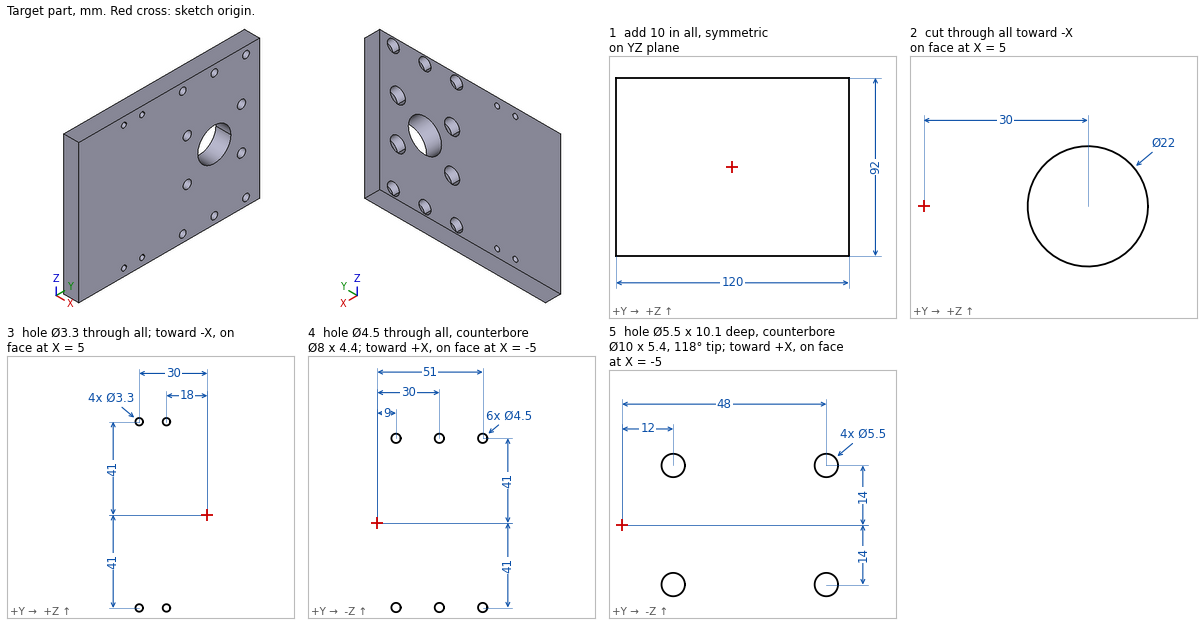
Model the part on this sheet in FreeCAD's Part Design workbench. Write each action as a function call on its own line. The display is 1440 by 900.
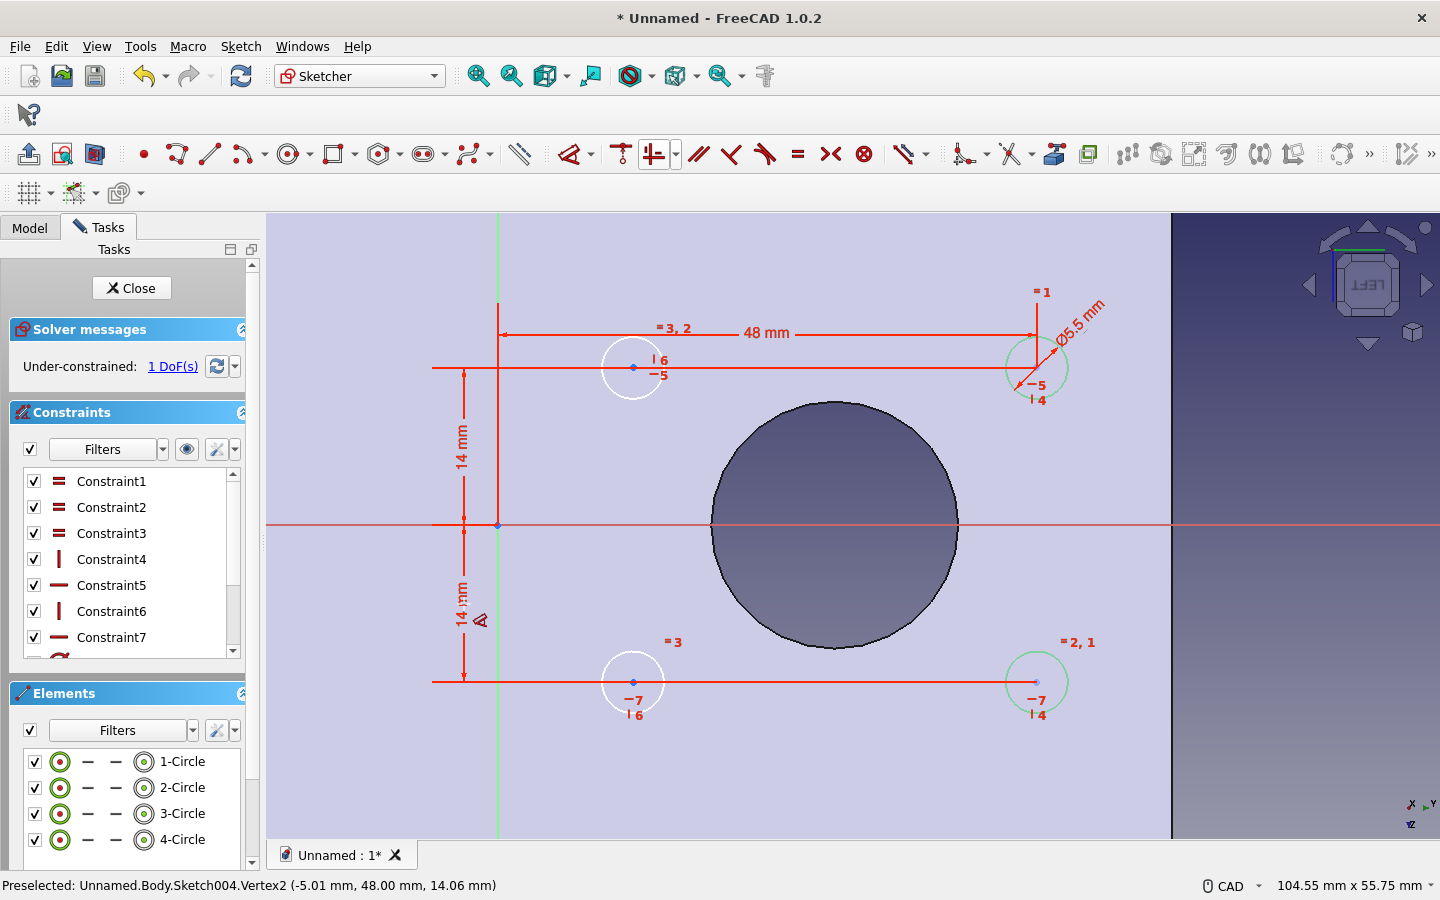
click(633, 368)
click(565, 334)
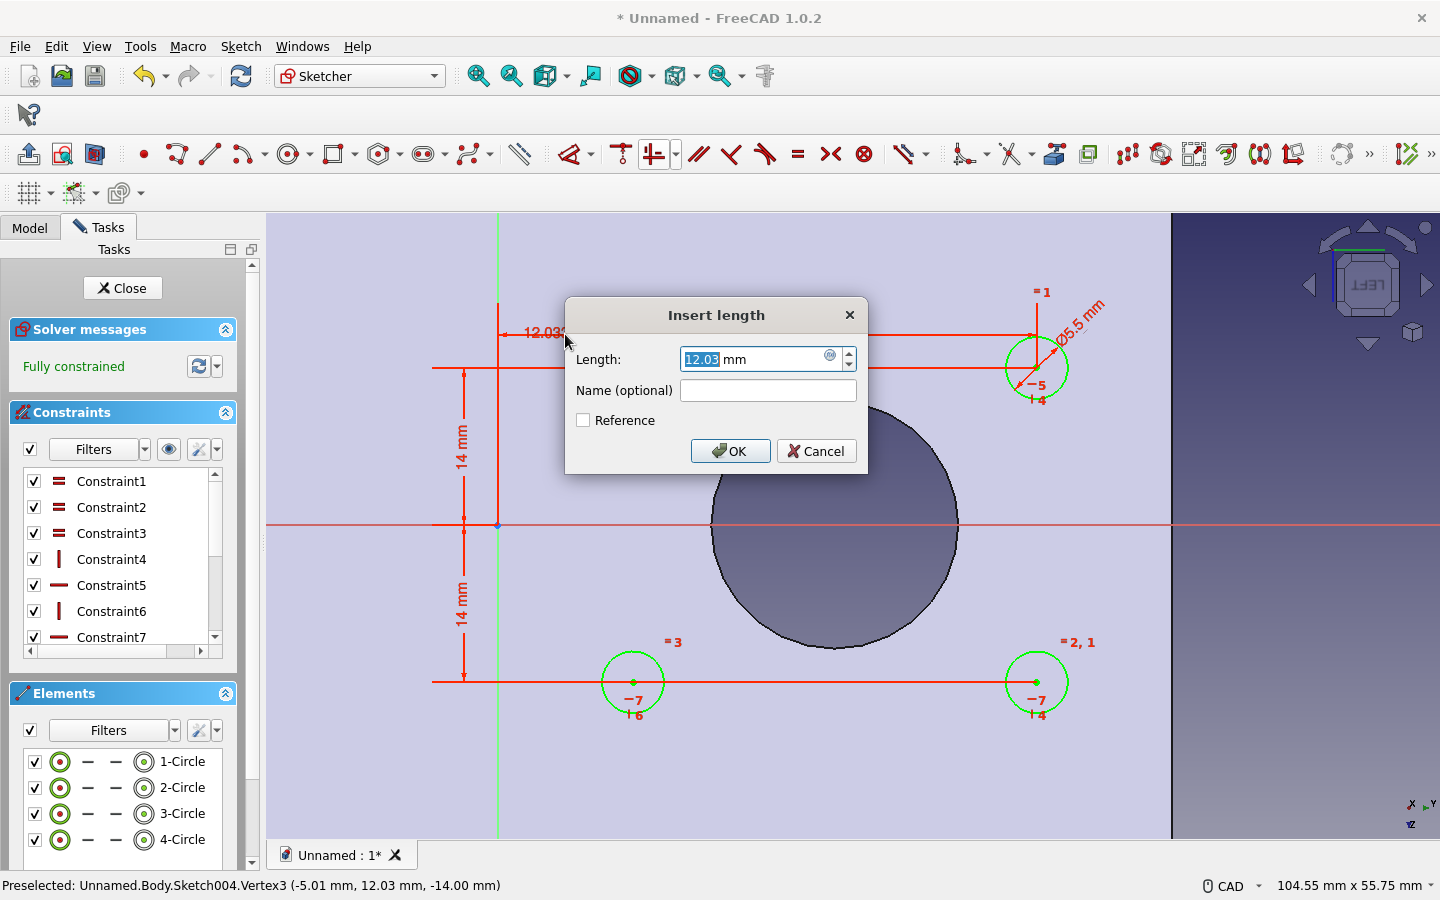
text(12)
key(Return)
key(Escape)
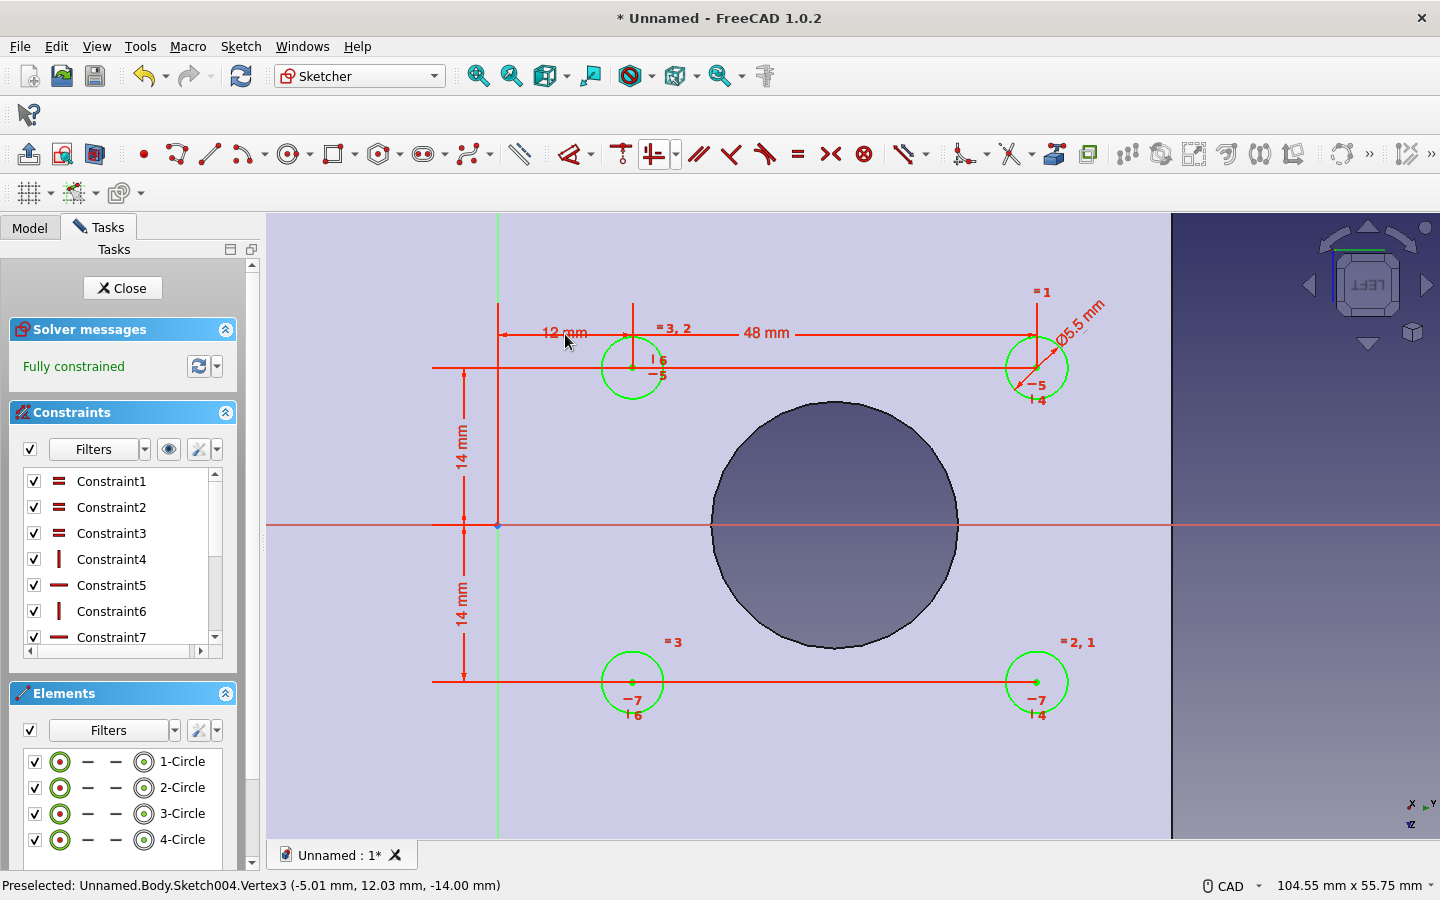
click(123, 288)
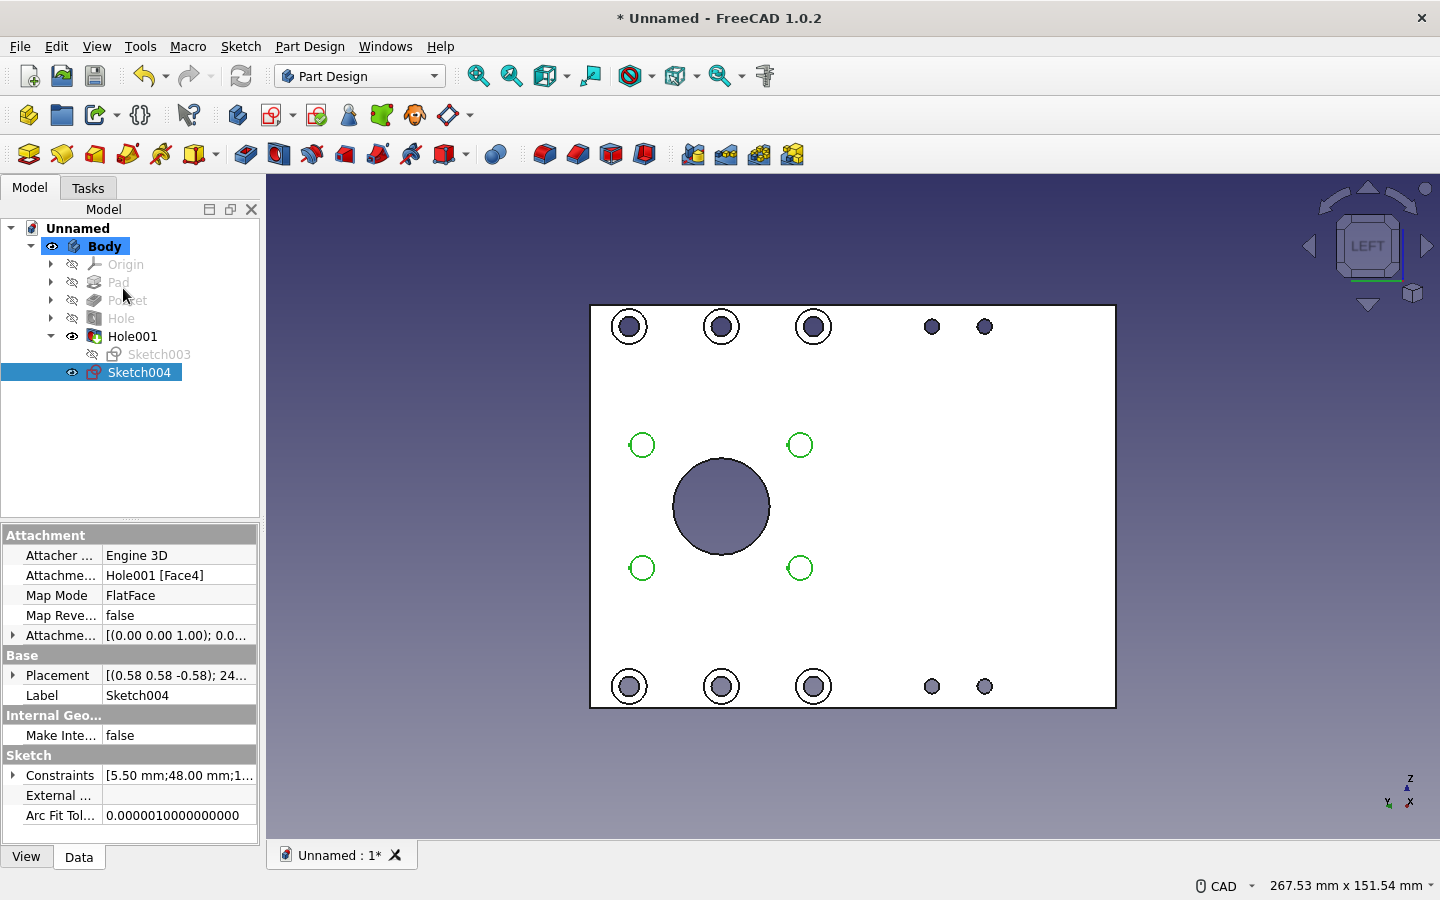
click(279, 154)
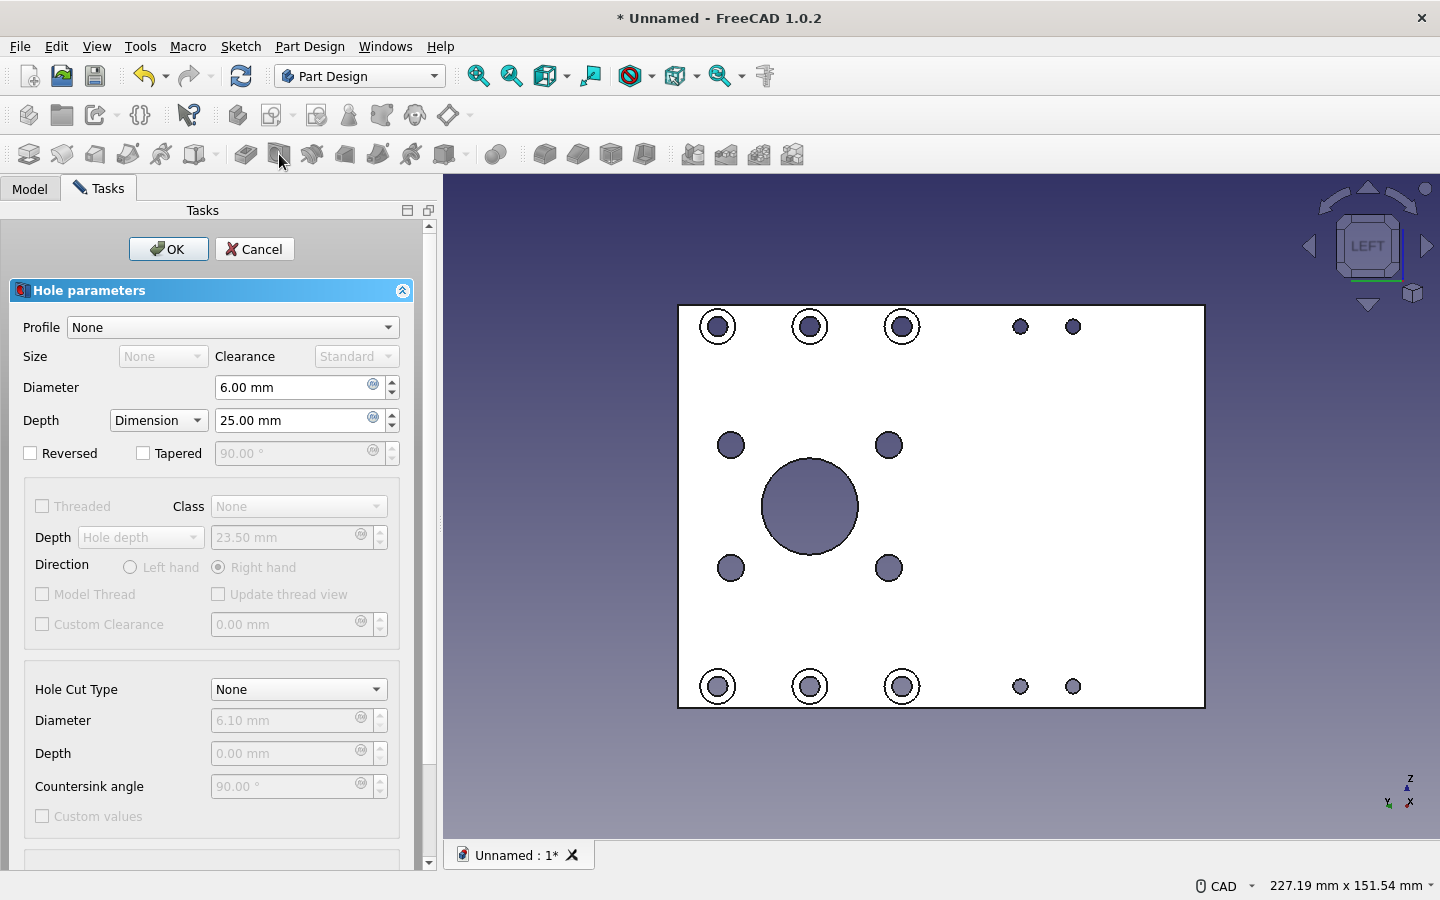
triple_click(300, 388)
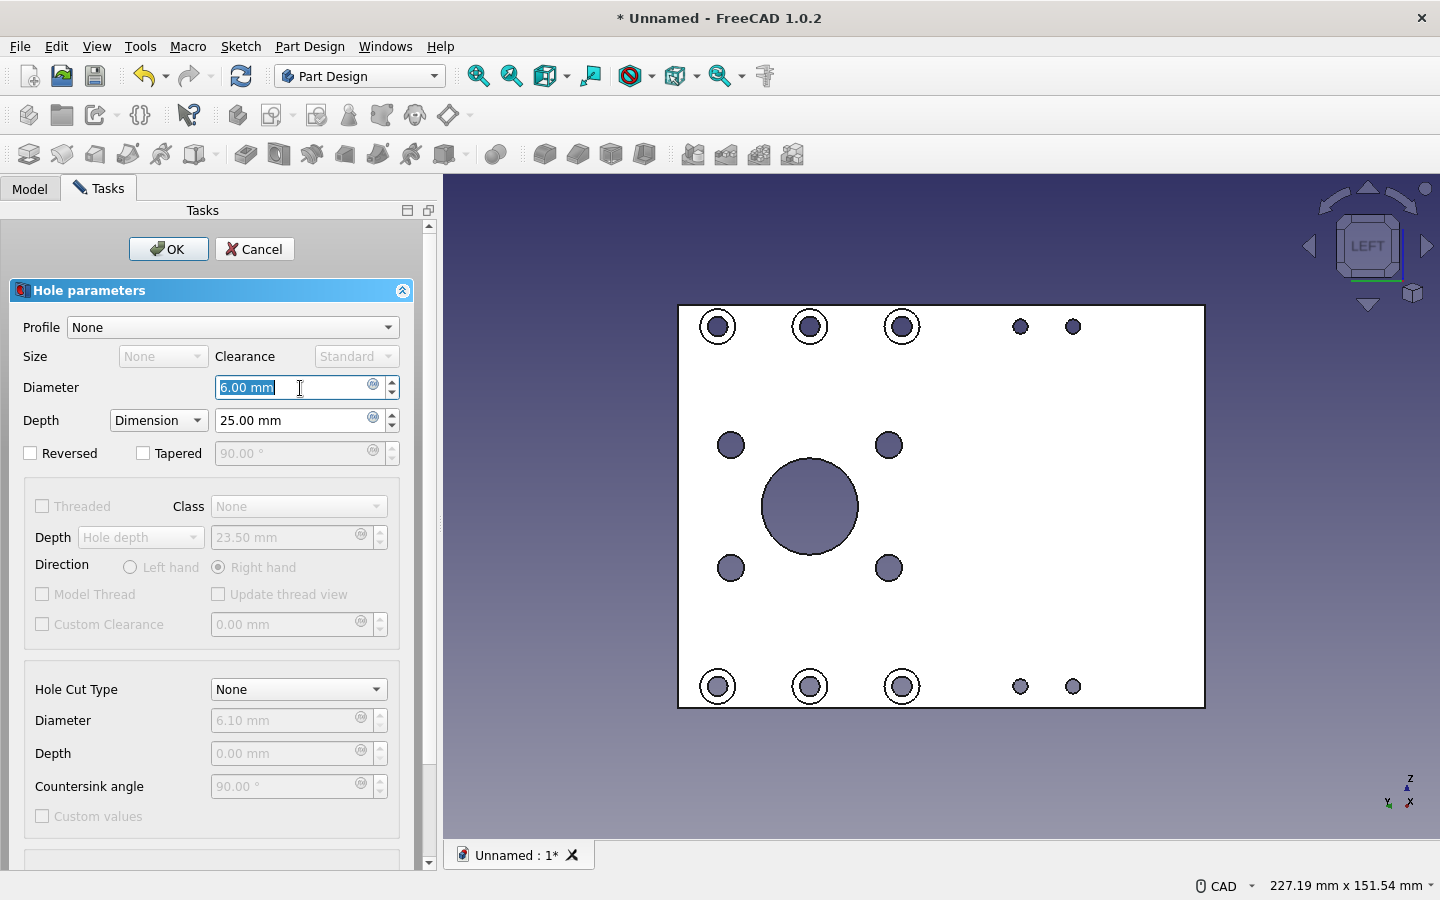
text(5.5)
key(Tab)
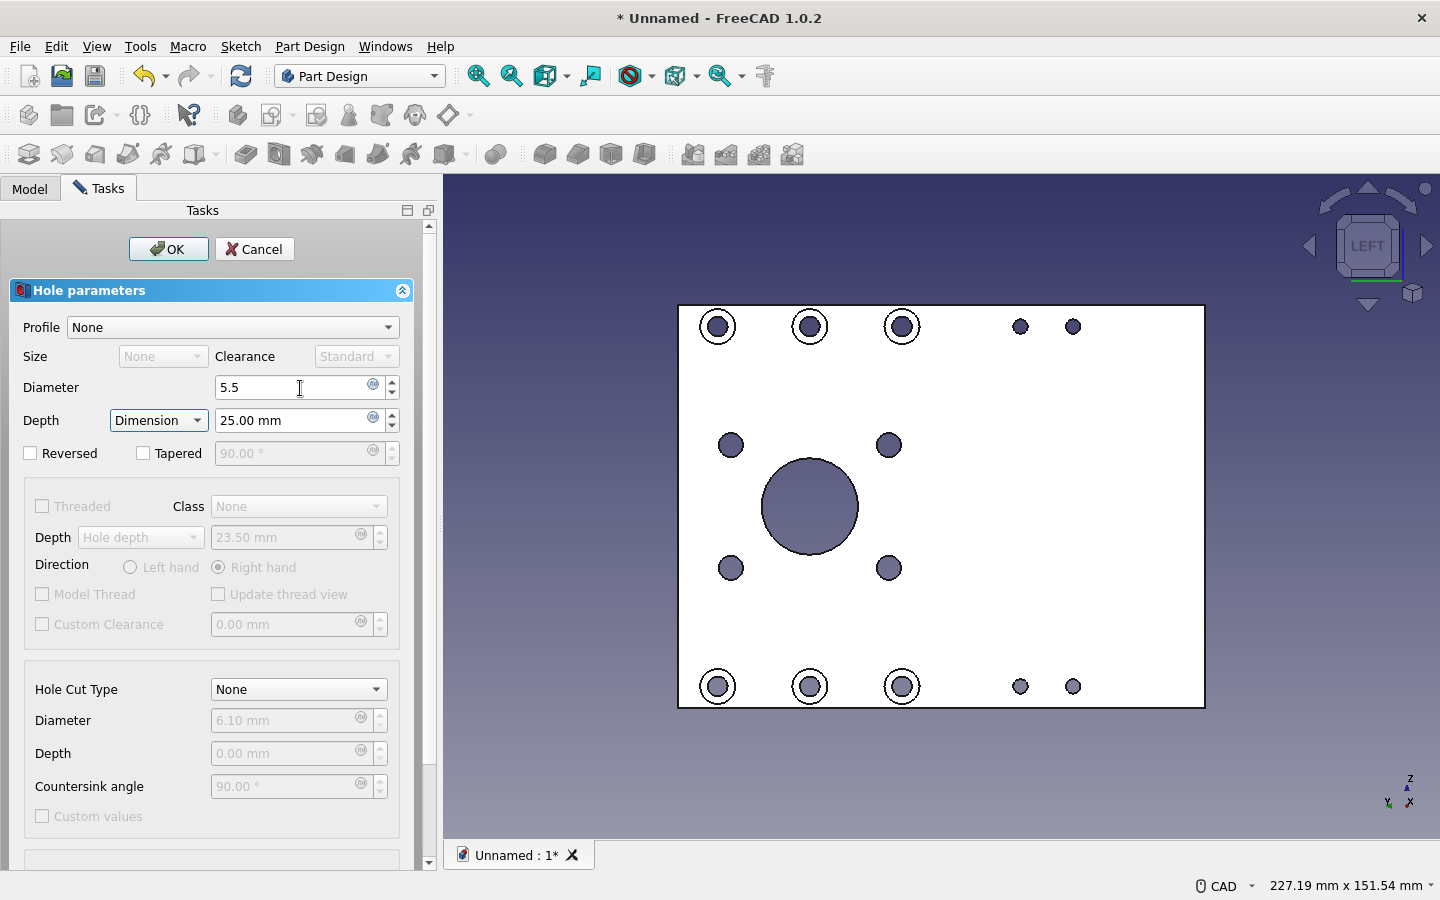
triple_click(300, 420)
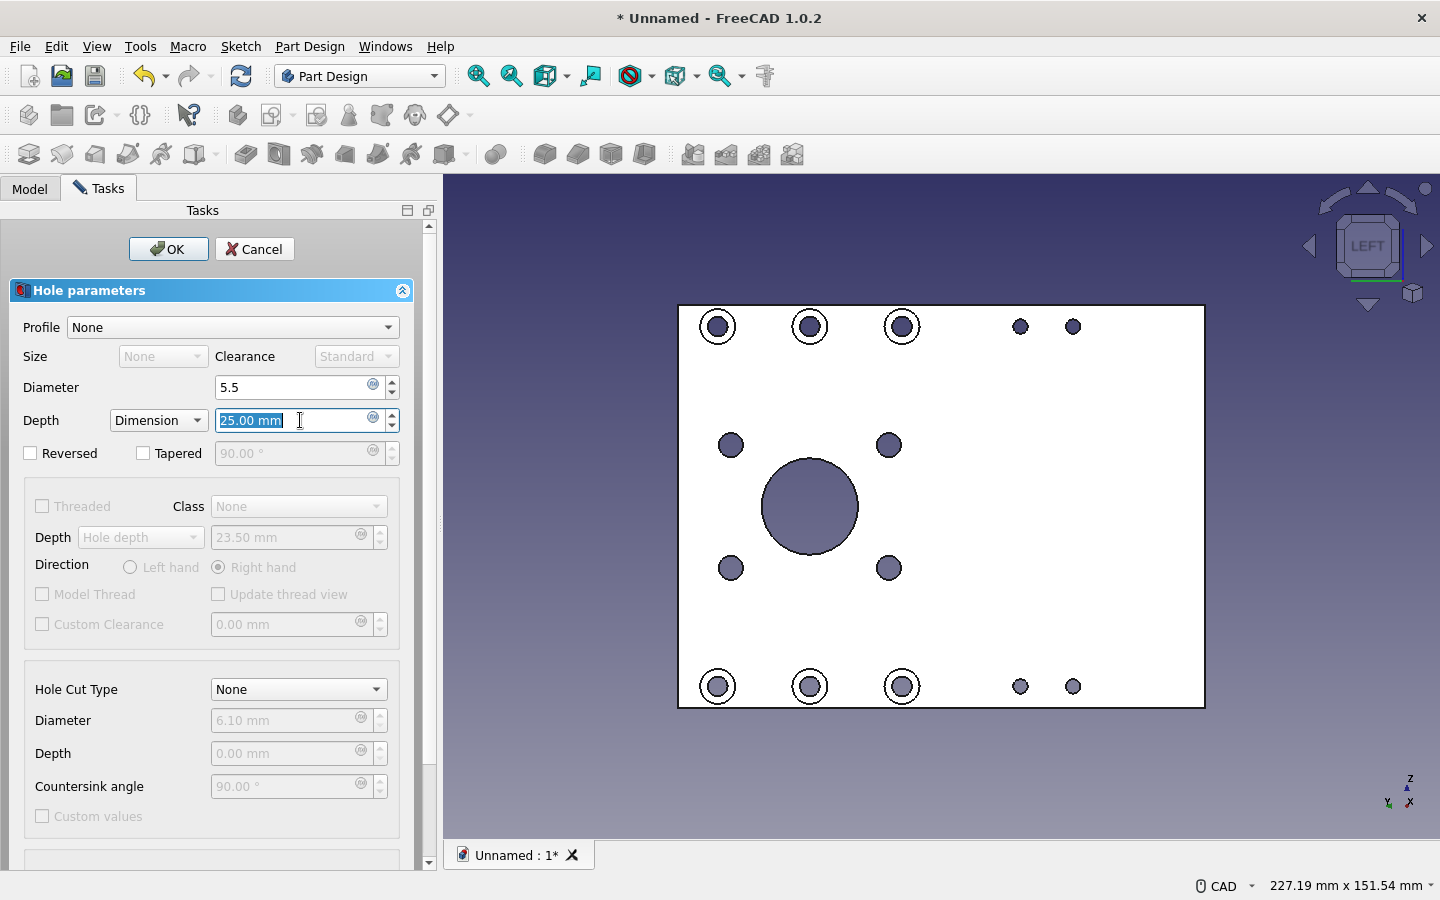
text(10.1)
key(Tab)